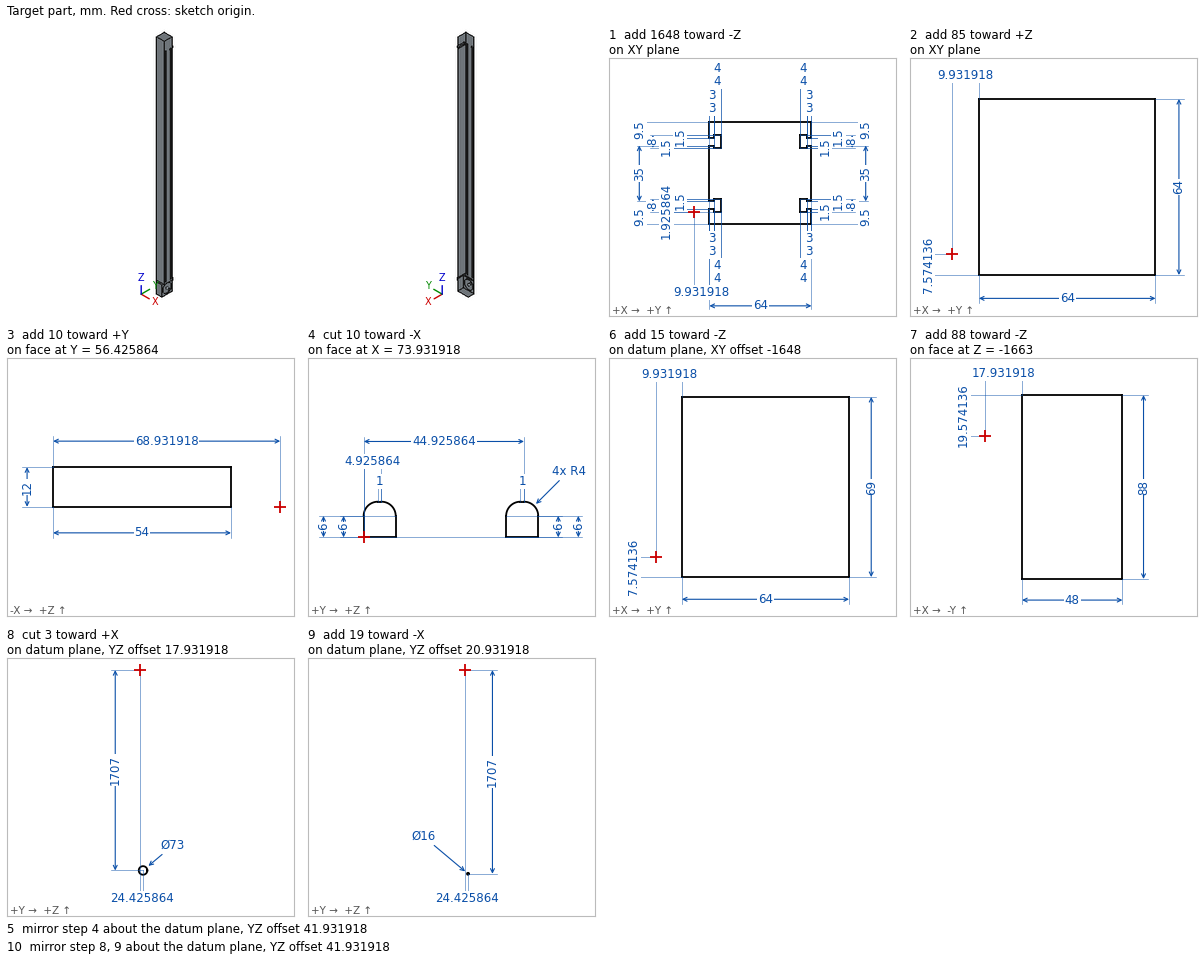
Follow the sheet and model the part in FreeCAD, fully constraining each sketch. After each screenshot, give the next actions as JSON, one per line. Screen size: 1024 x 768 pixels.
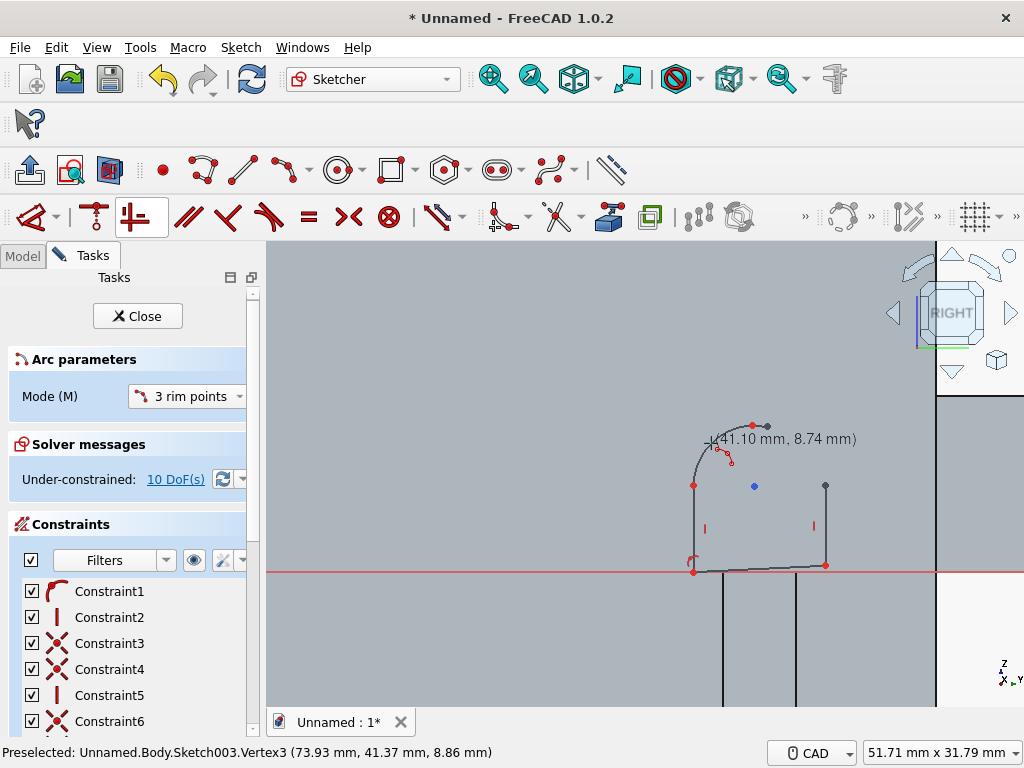
{"action": "left_click", "coordinate": [826, 485]}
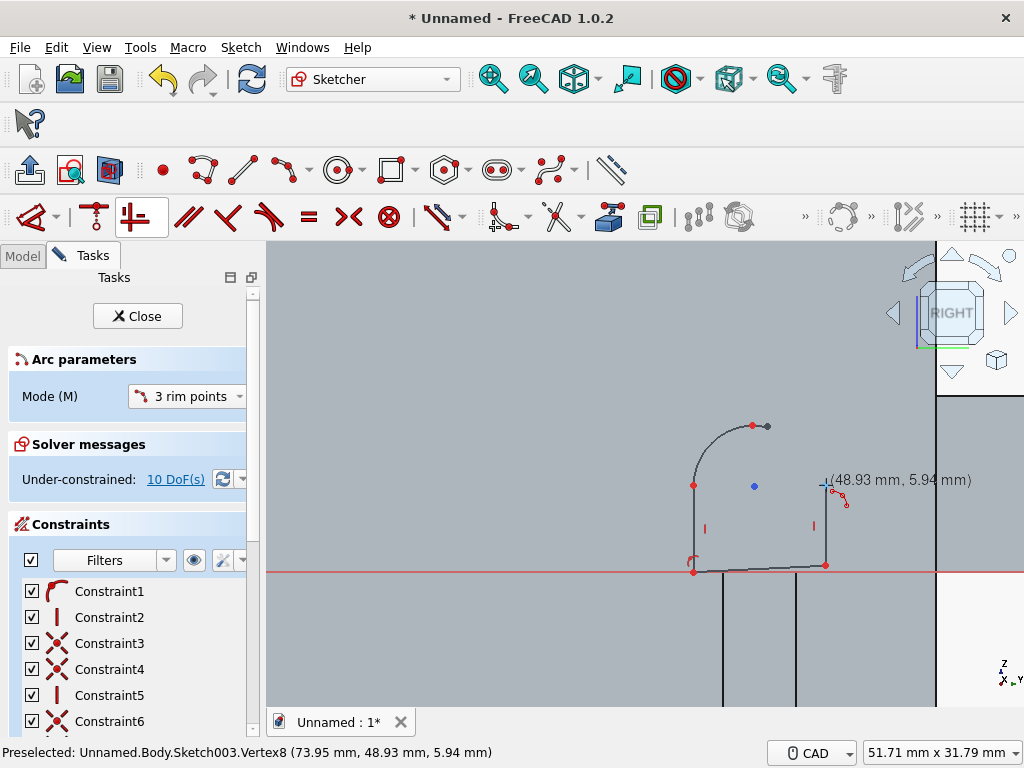
{"action": "scroll", "coordinate": [767, 426], "scroll_direction": "up", "scroll_amount": 4}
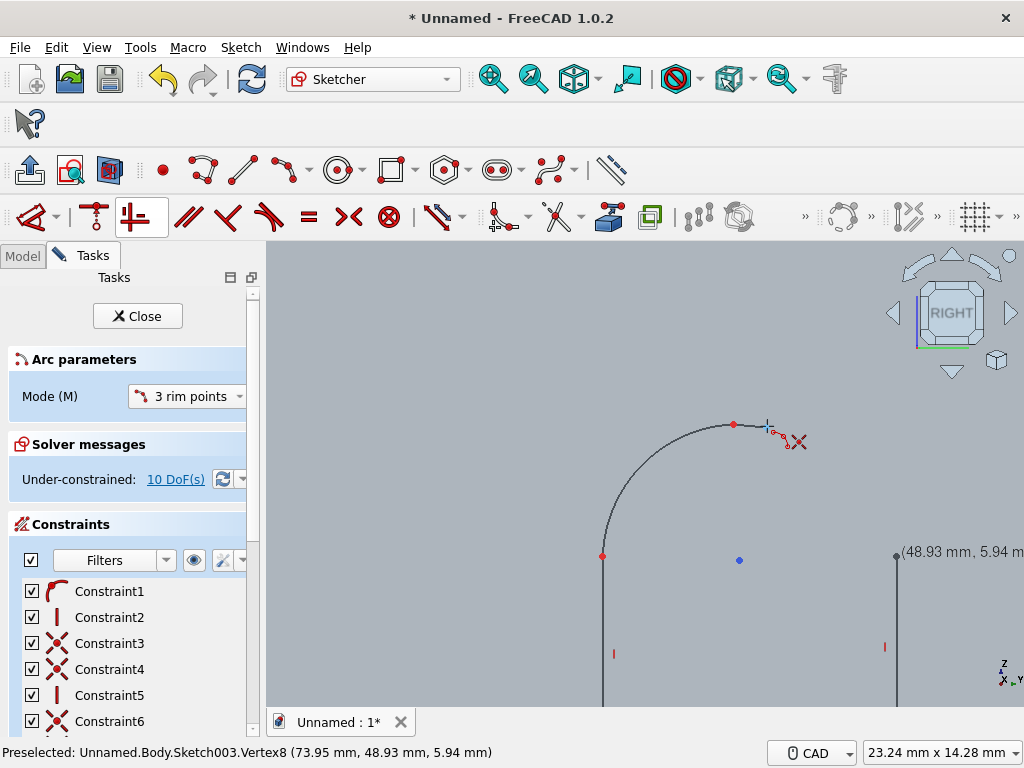
{"action": "left_click", "coordinate": [766, 428]}
{"action": "left_click", "coordinate": [858, 463]}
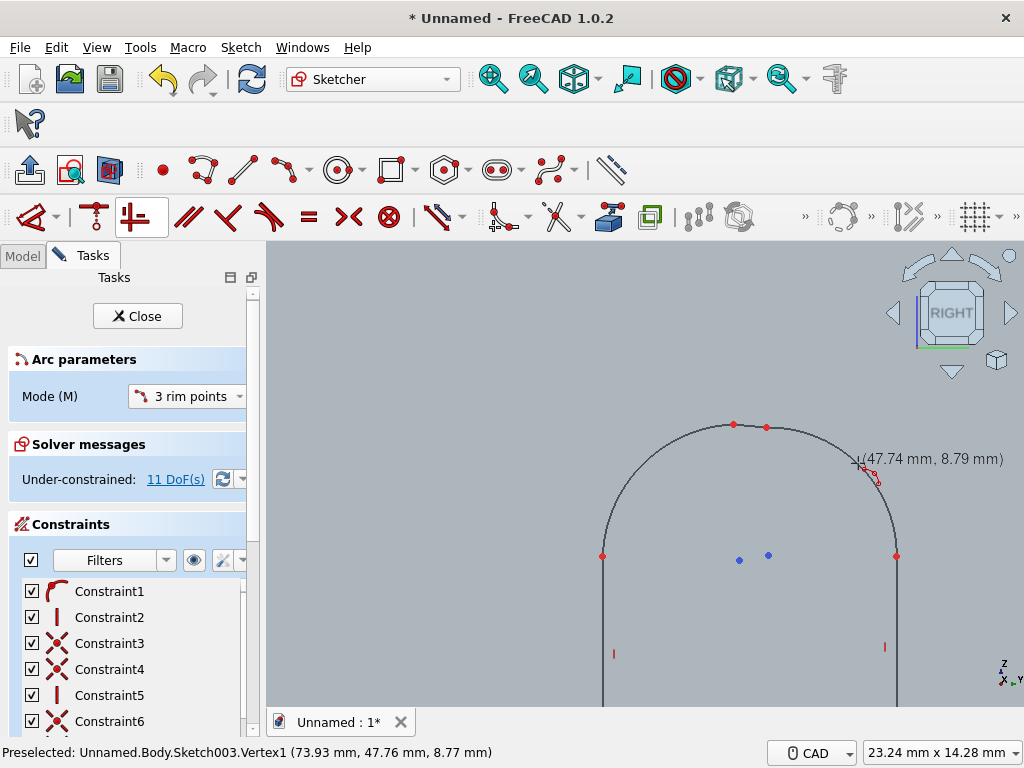
{"action": "left_click", "coordinate": [244, 170]}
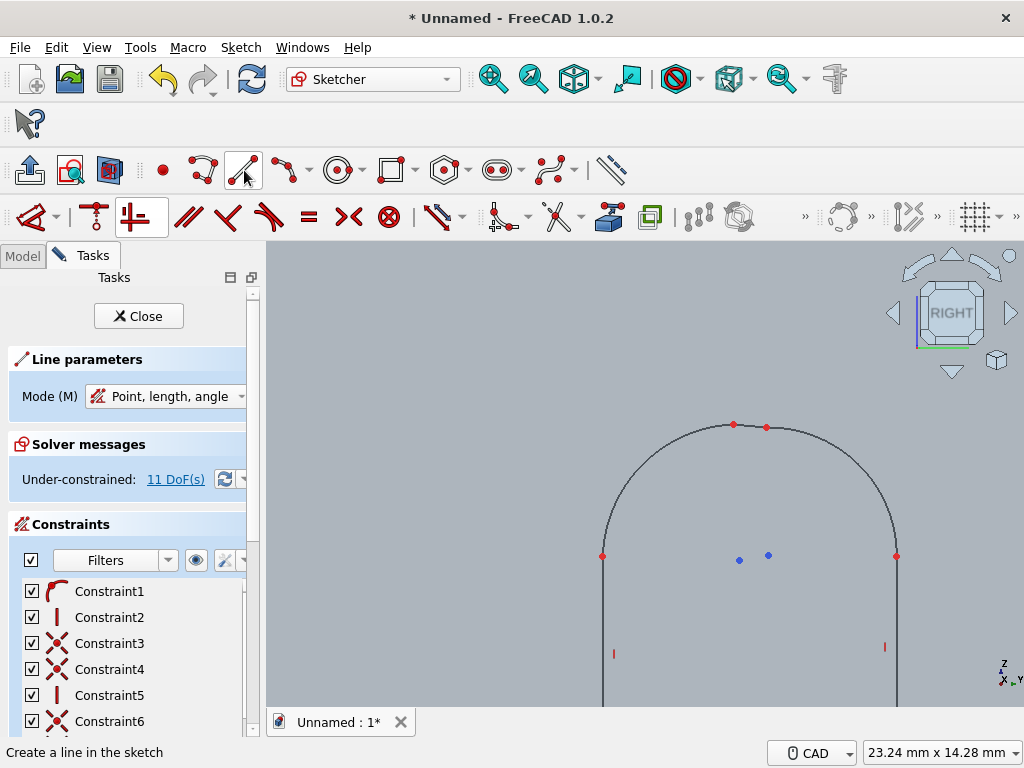
{"action": "scroll", "coordinate": [733, 437], "scroll_direction": "down", "scroll_amount": 7}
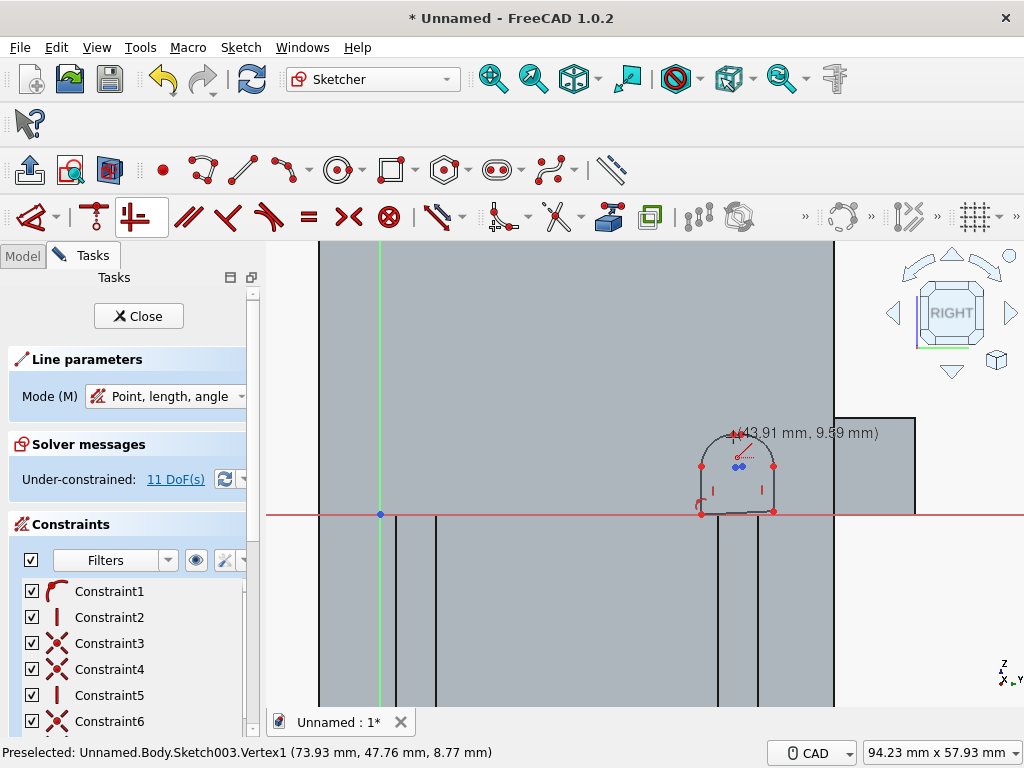
{"action": "left_click", "coordinate": [420, 434]}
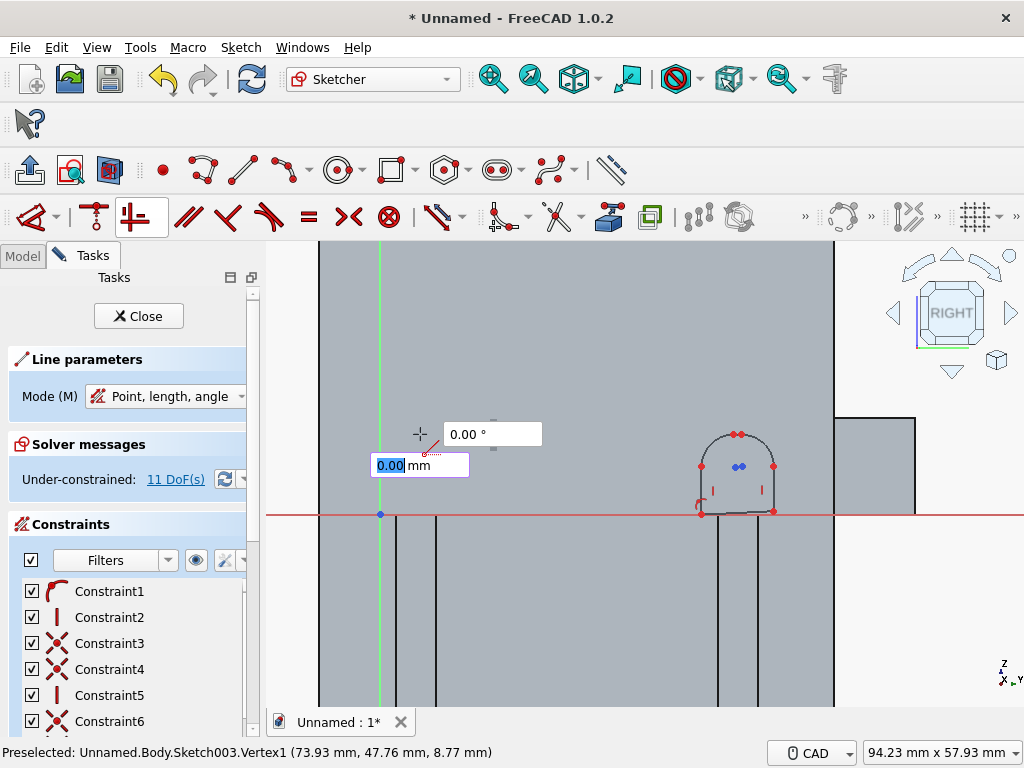
{"action": "scroll", "coordinate": [412, 434], "scroll_direction": "up", "scroll_amount": 4}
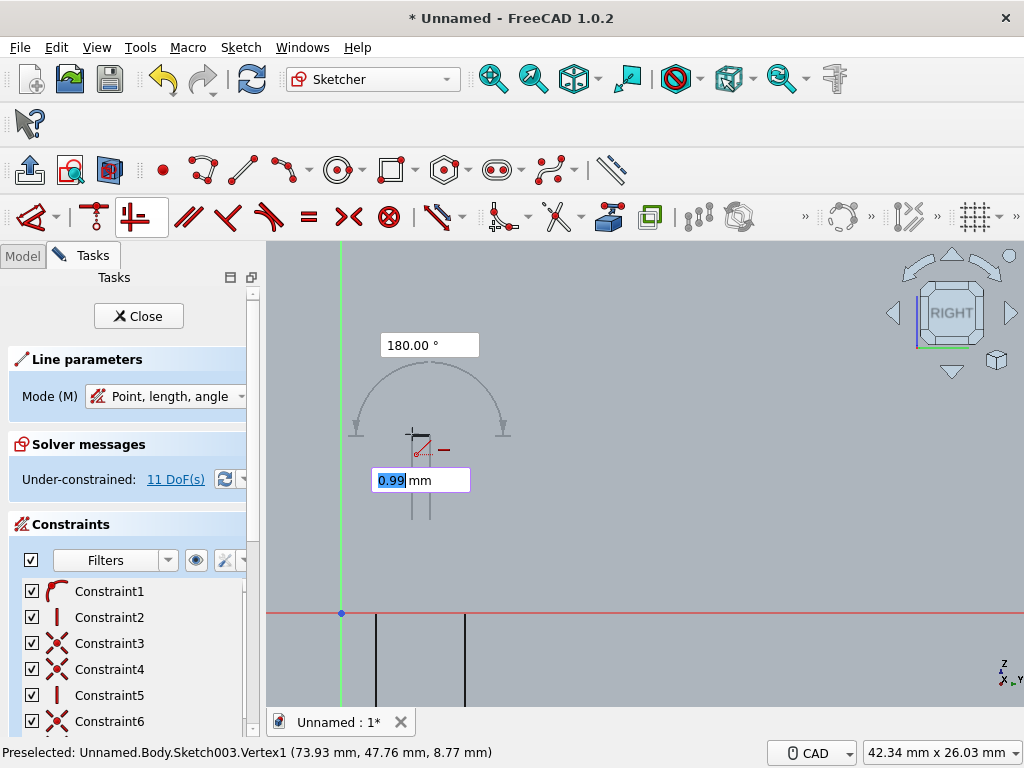
{"action": "left_click", "coordinate": [411, 433]}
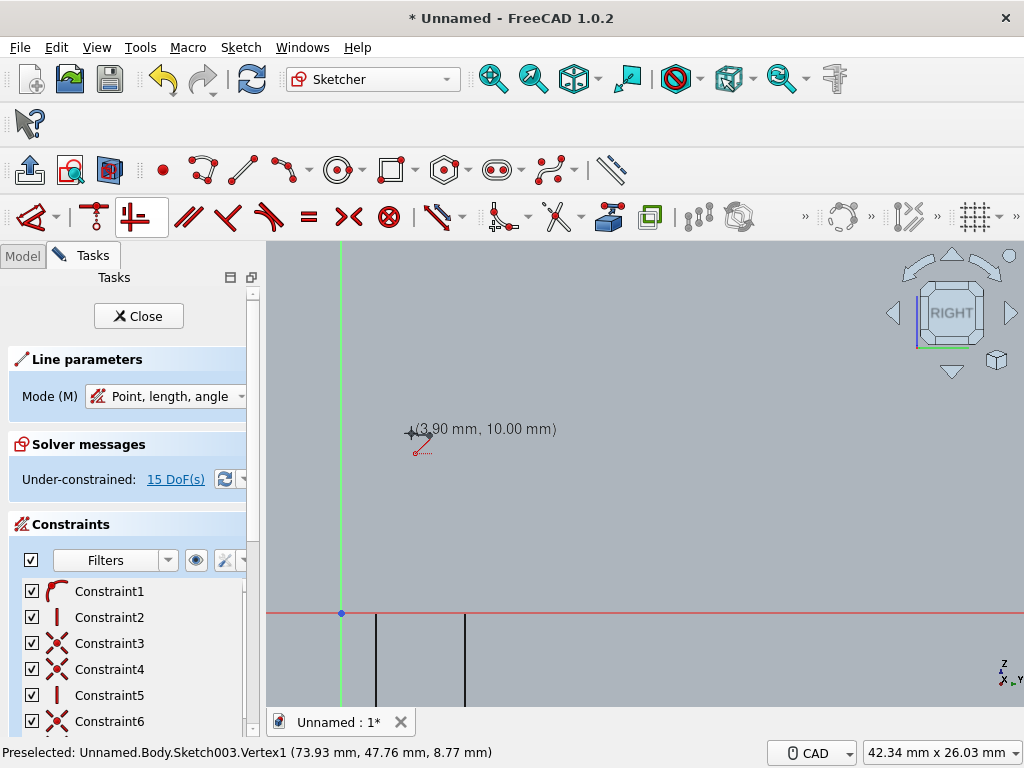
{"action": "left_click", "coordinate": [204, 170]}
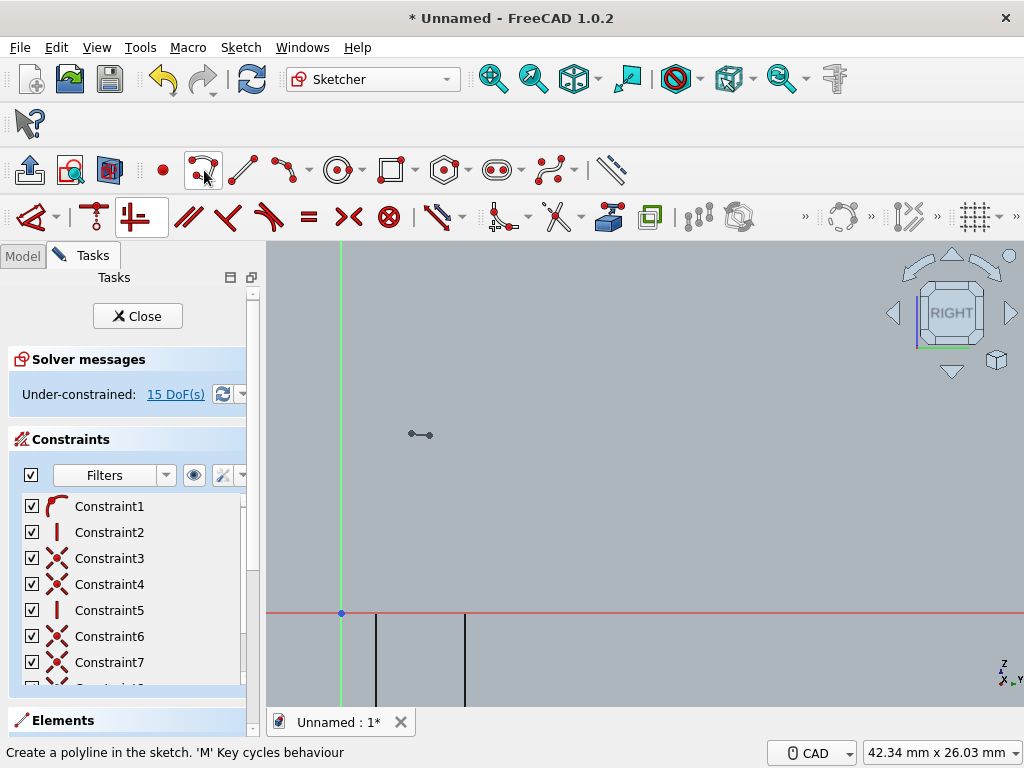
{"action": "scroll", "coordinate": [340, 506], "scroll_direction": "up", "scroll_amount": 13}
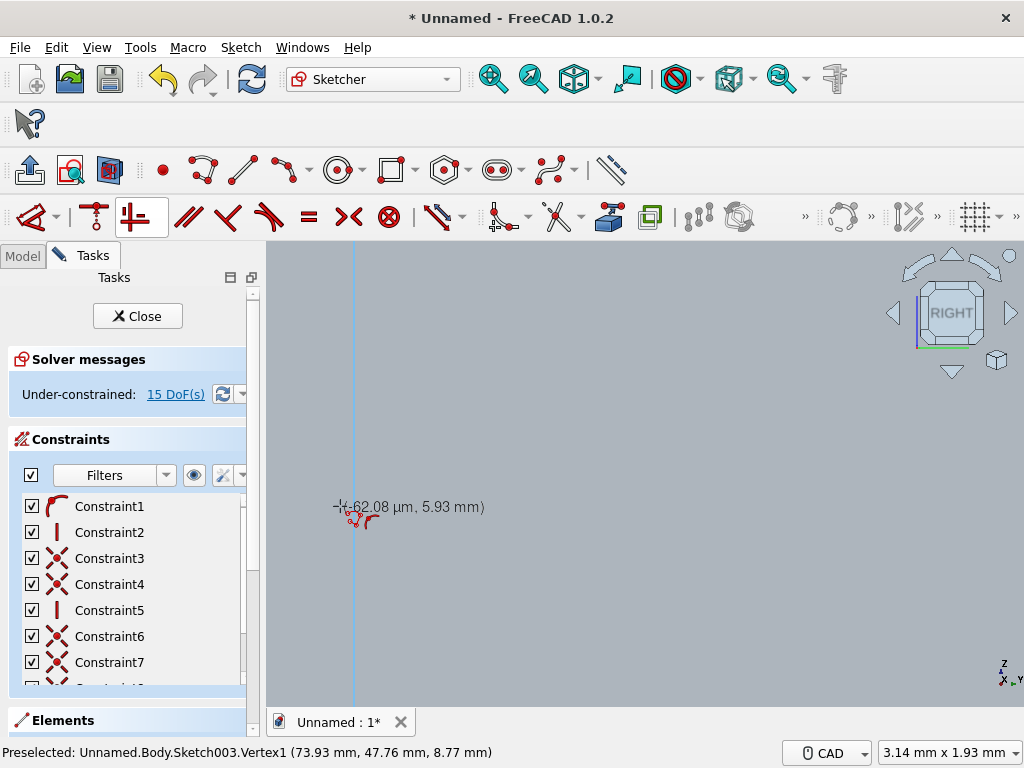
{"action": "left_click", "coordinate": [336, 494]}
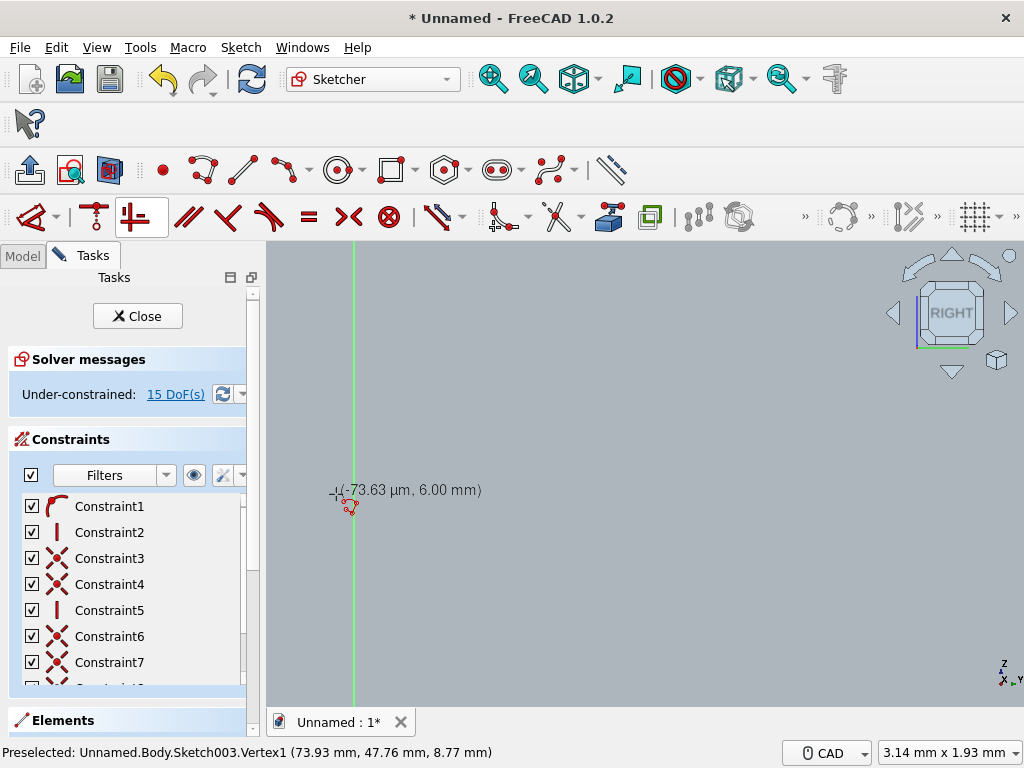
{"action": "scroll", "coordinate": [336, 463], "scroll_direction": "down", "scroll_amount": 16}